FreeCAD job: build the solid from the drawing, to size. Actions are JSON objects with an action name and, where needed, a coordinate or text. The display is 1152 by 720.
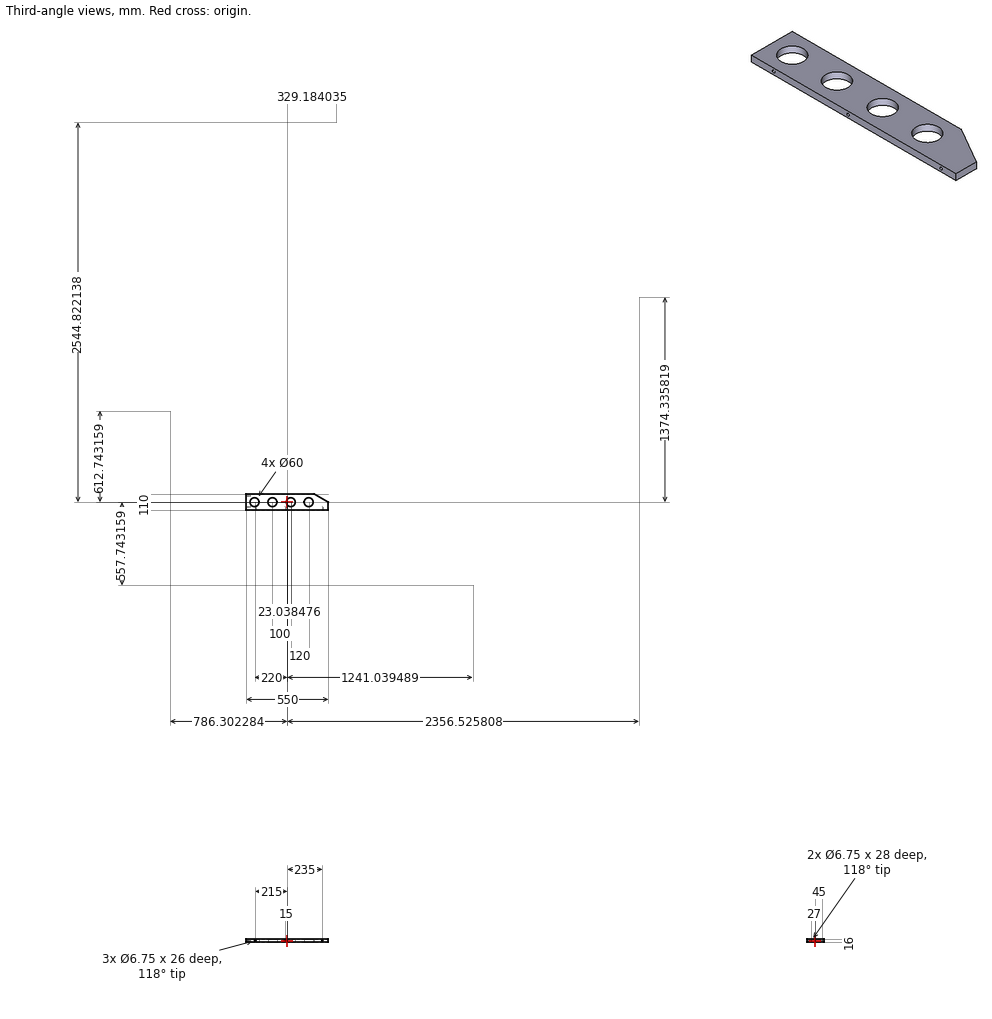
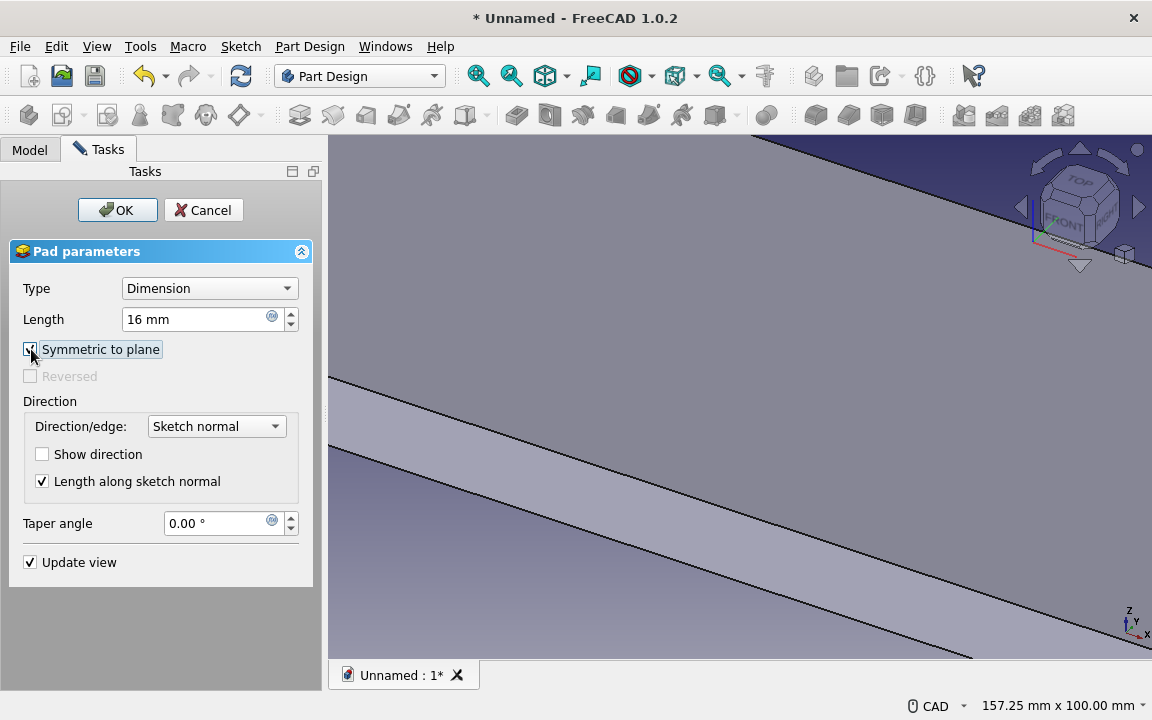
{"action": "left_click", "coordinate": [118, 210]}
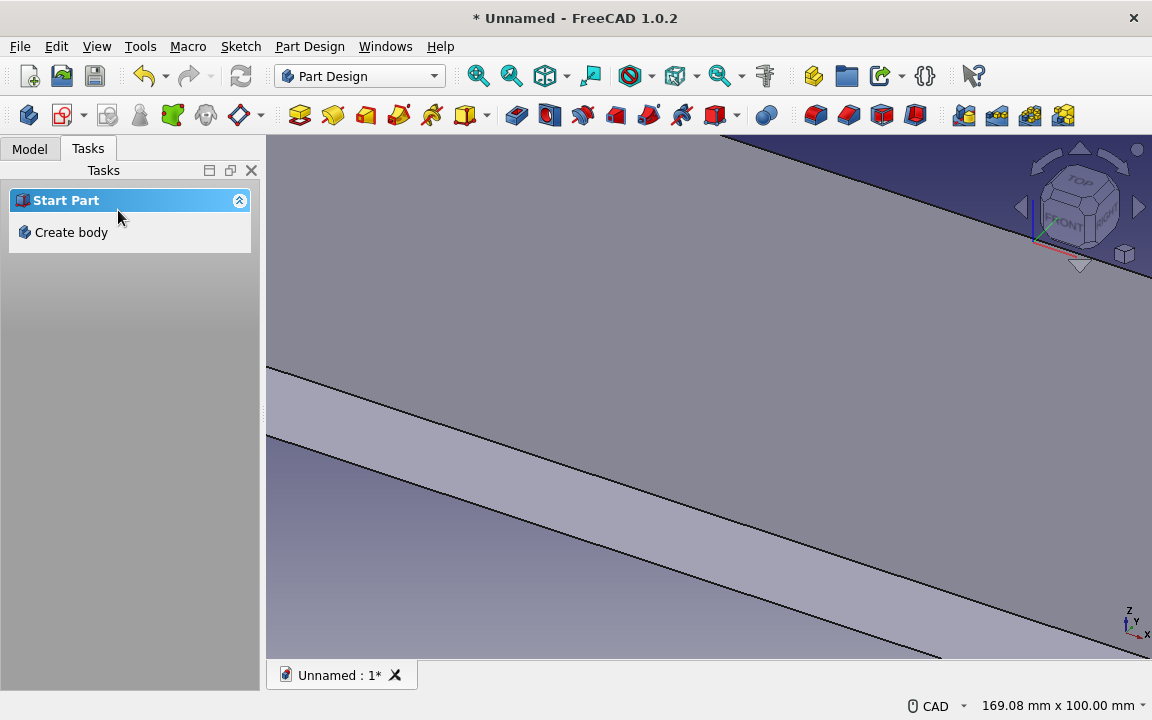
{"action": "key", "text": "v f"}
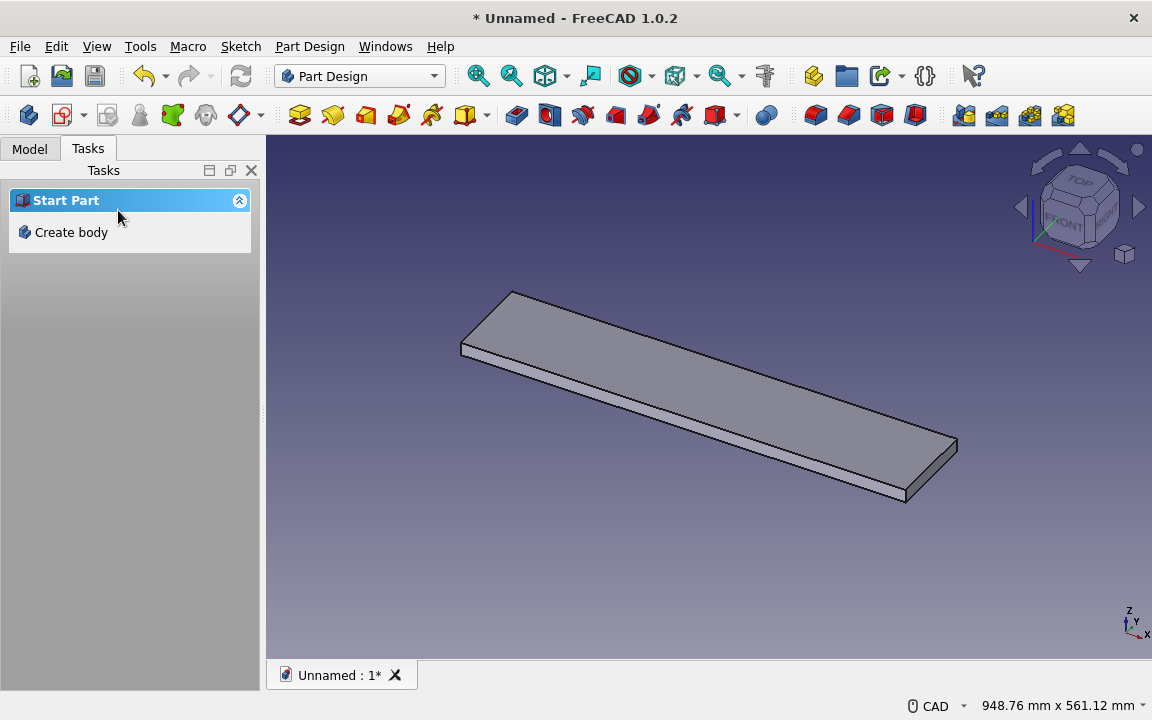
{"action": "left_click", "coordinate": [836, 432]}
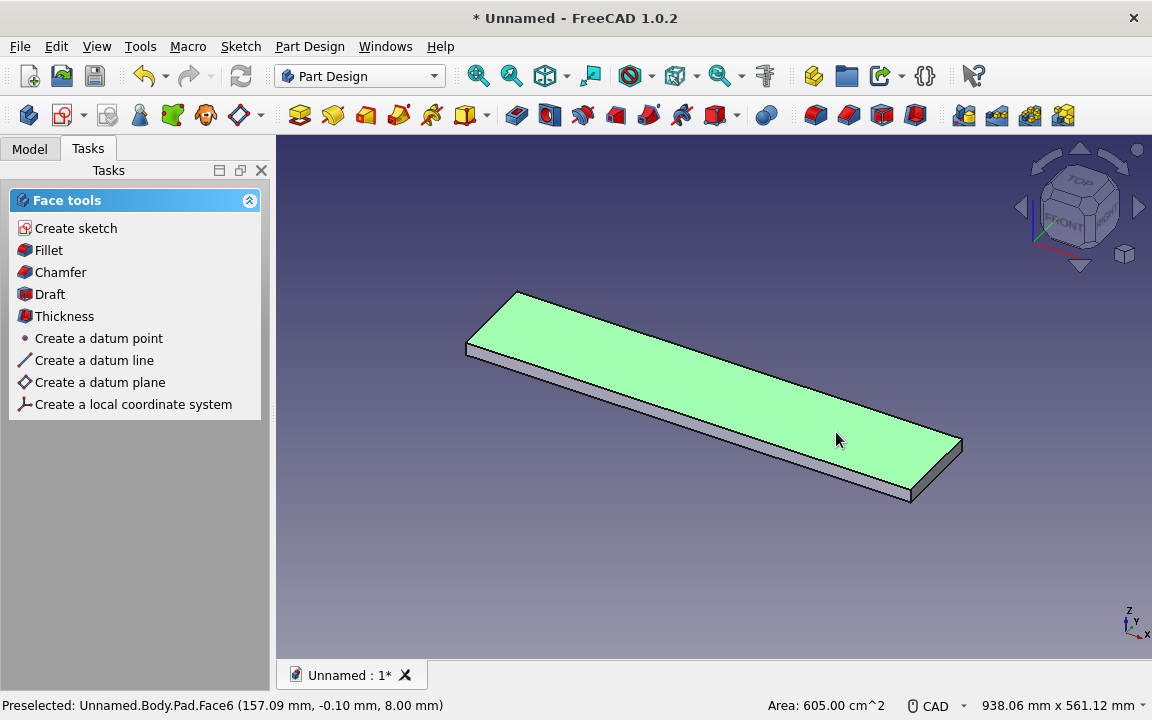
{"action": "left_click", "coordinate": [62, 116]}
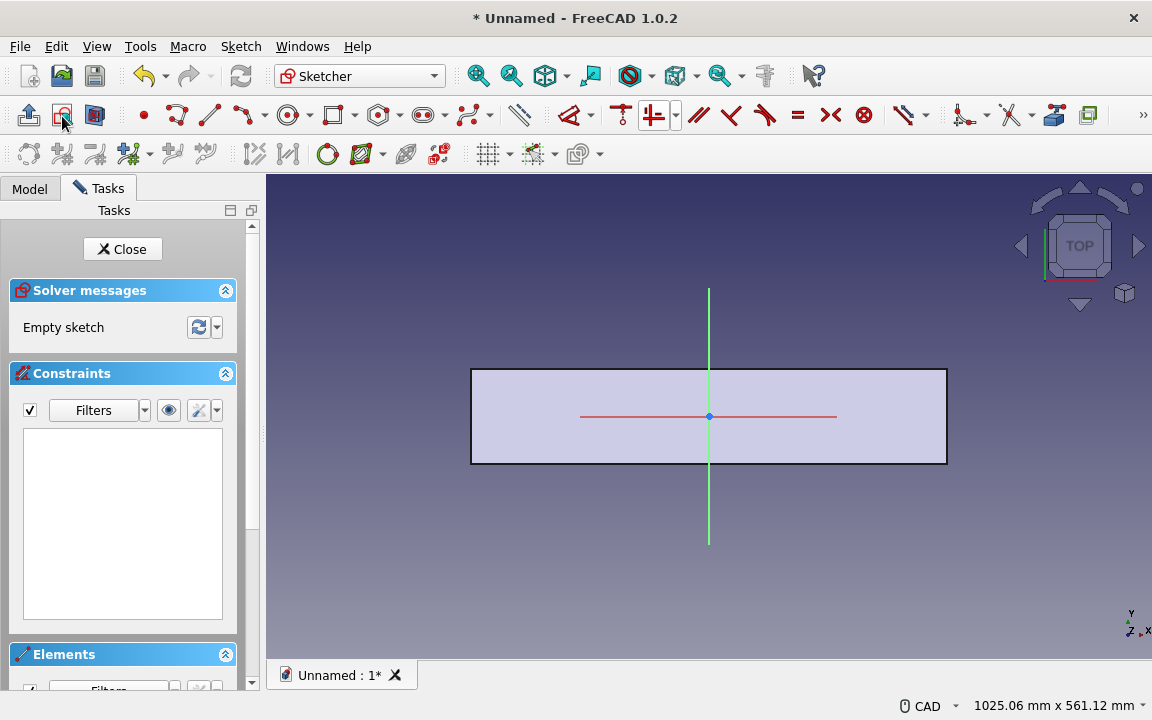
{"action": "scroll", "coordinate": [547, 524], "scroll_direction": "down", "scroll_amount": 11}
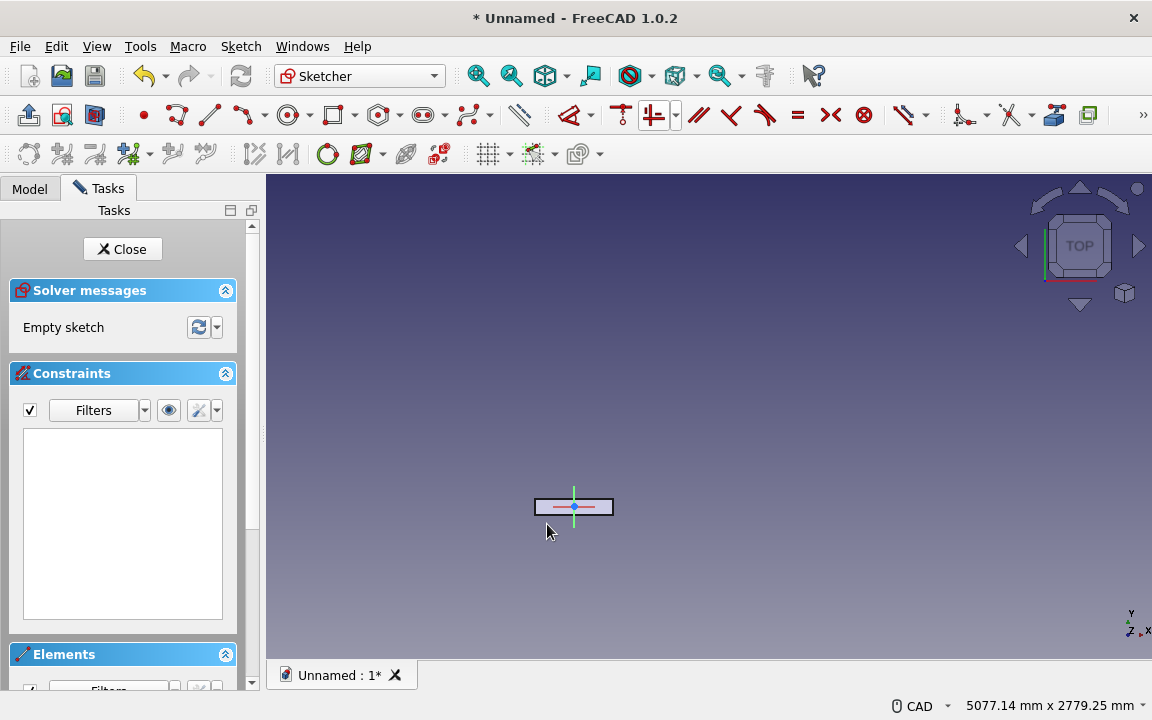
{"action": "left_click", "coordinate": [177, 116]}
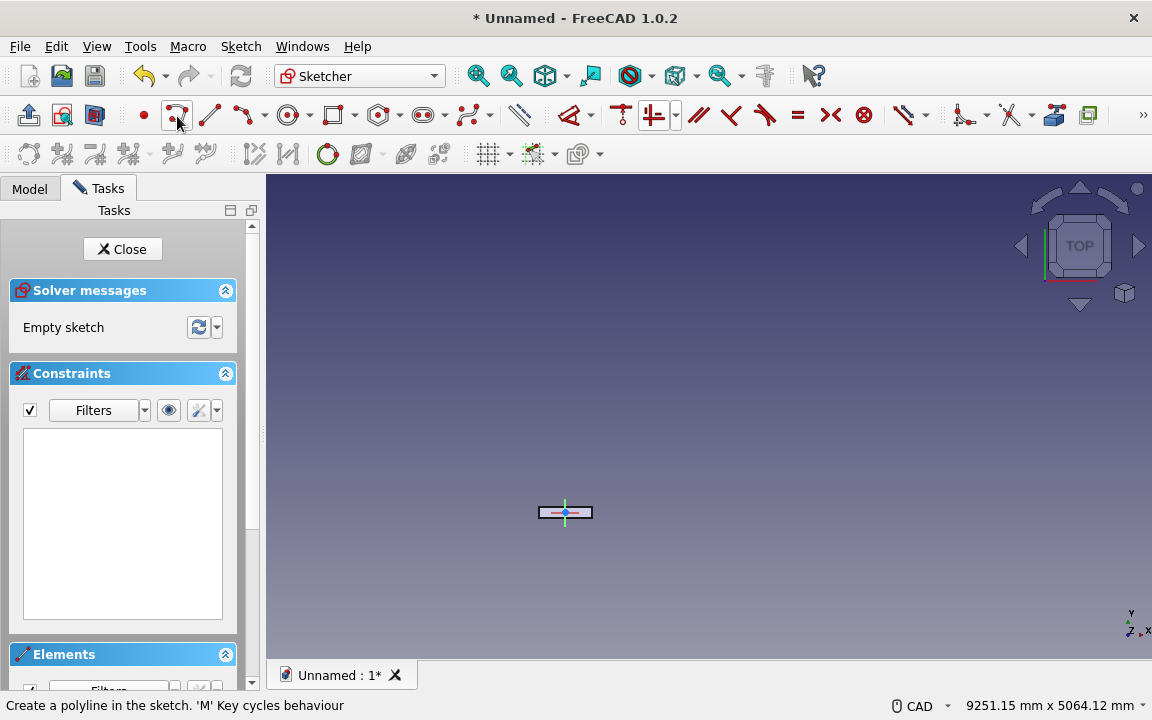
{"action": "left_click", "coordinate": [490, 454]}
{"action": "left_click", "coordinate": [684, 566]}
{"action": "left_click", "coordinate": [791, 381]}
{"action": "left_click", "coordinate": [597, 269]}
{"action": "left_click", "coordinate": [490, 455]}
{"action": "key", "text": "Escape"}
{"action": "key", "text": "Escape"}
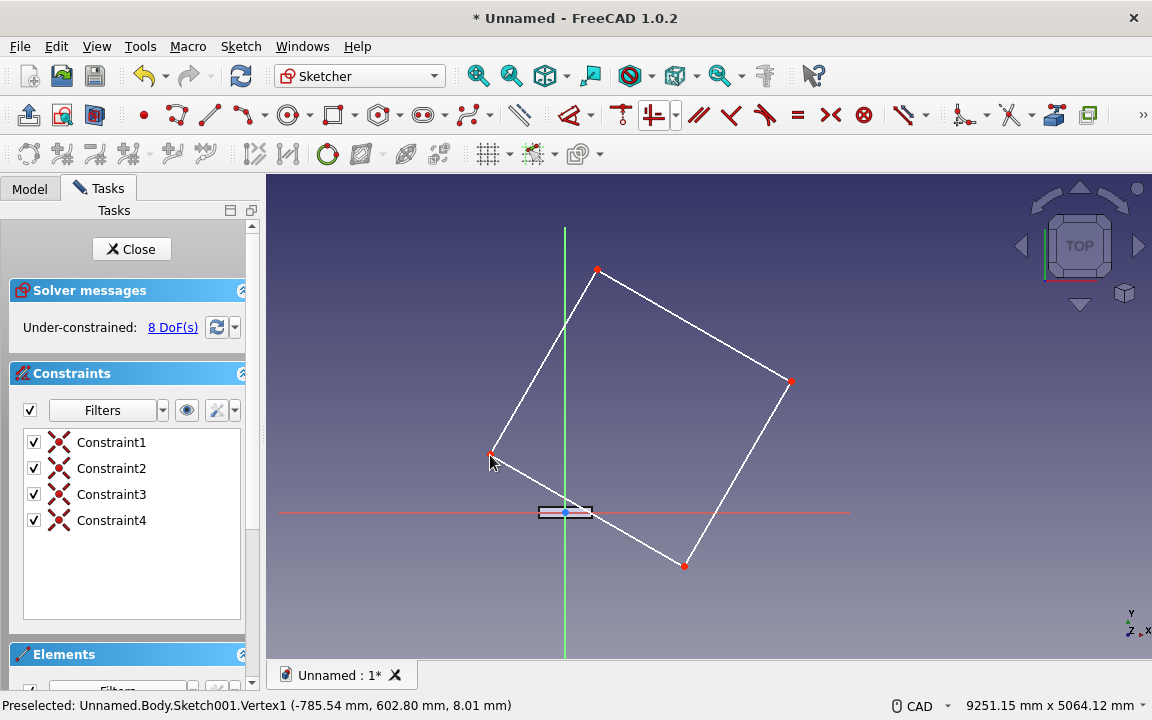
{"action": "key", "text": "d"}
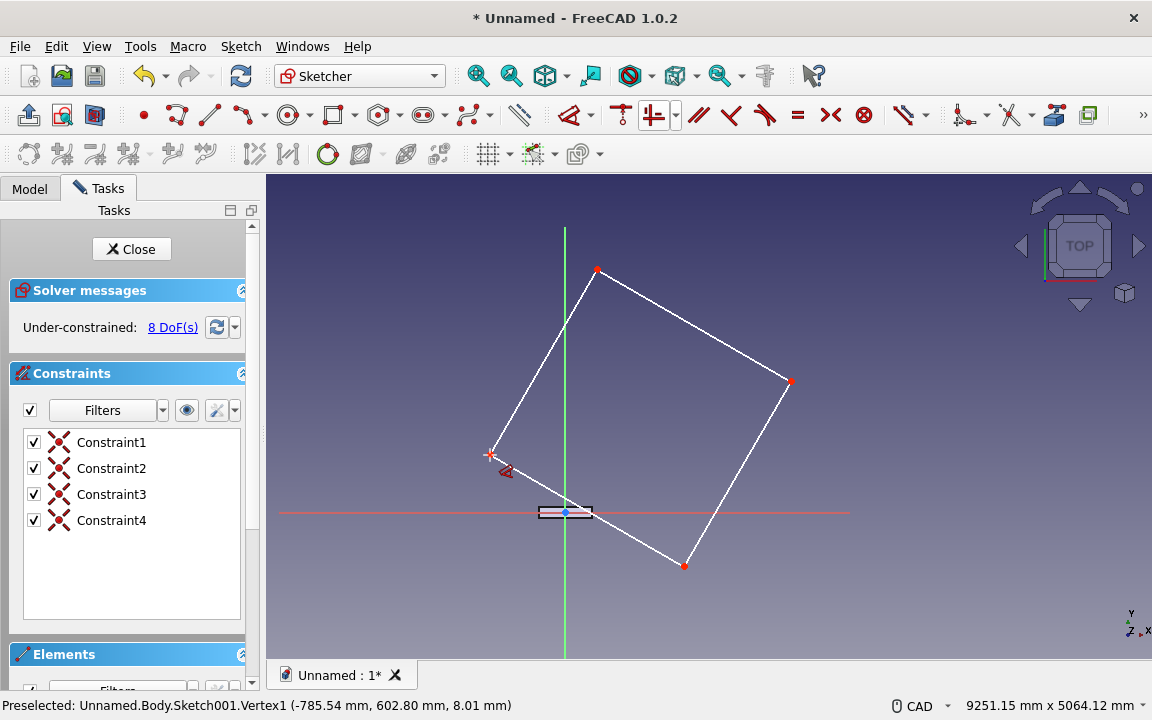
{"action": "left_click", "coordinate": [490, 455]}
{"action": "left_click", "coordinate": [528, 547]}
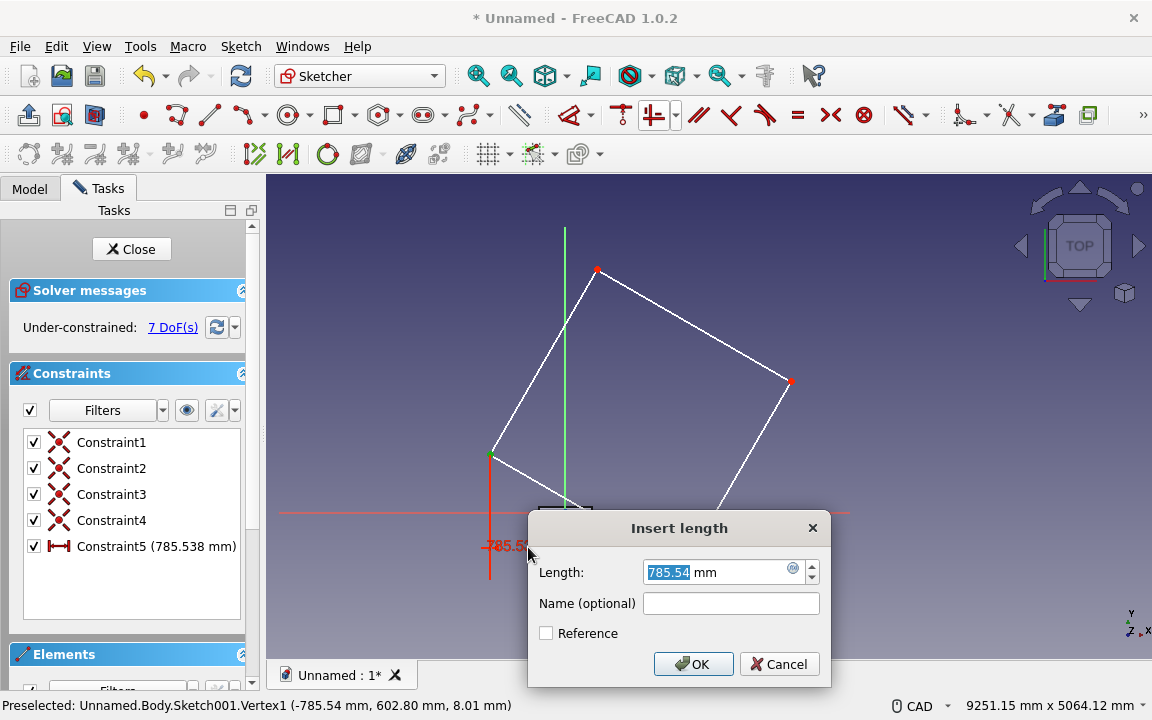
{"action": "type", "text": "786.302284"}
{"action": "key", "text": "Return"}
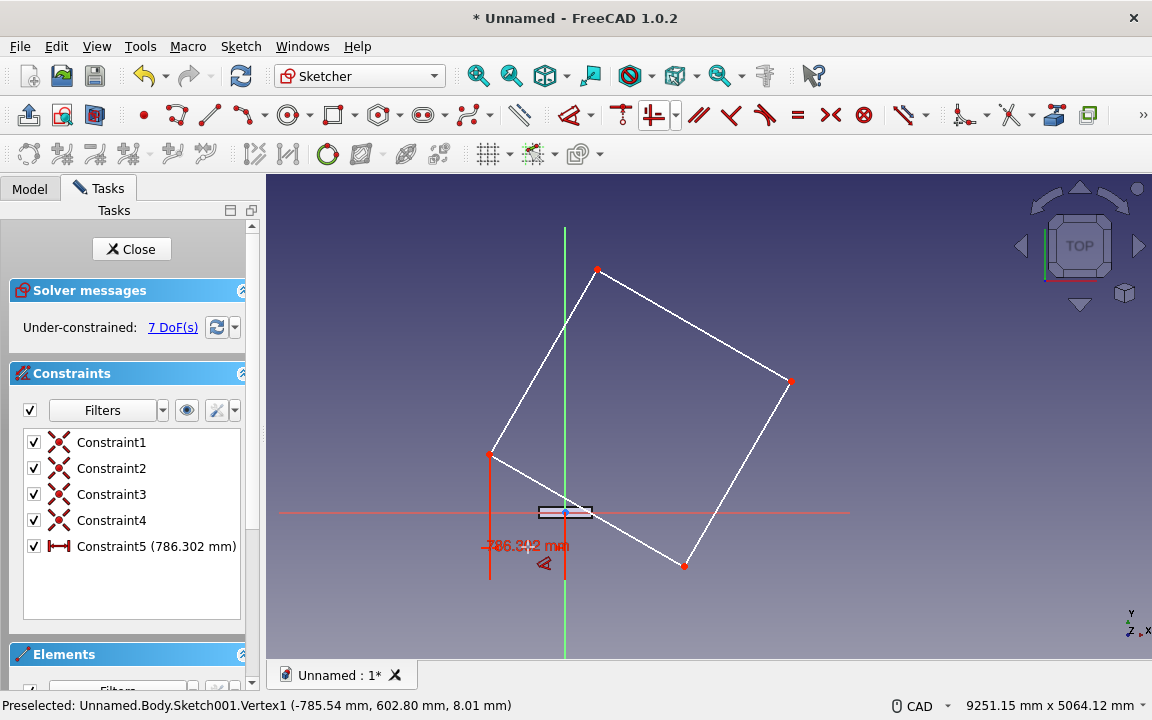
{"action": "left_click", "coordinate": [490, 455]}
{"action": "left_click", "coordinate": [456, 484]}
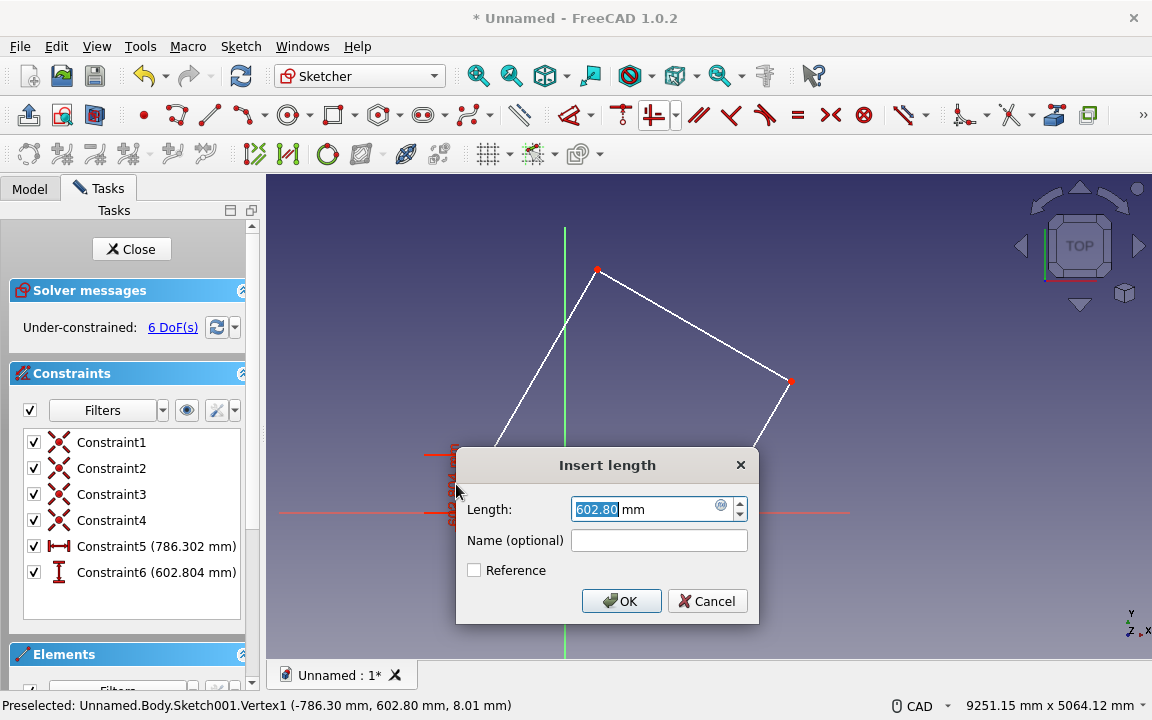
{"action": "type", "text": "612.743159"}
{"action": "key", "text": "Return"}